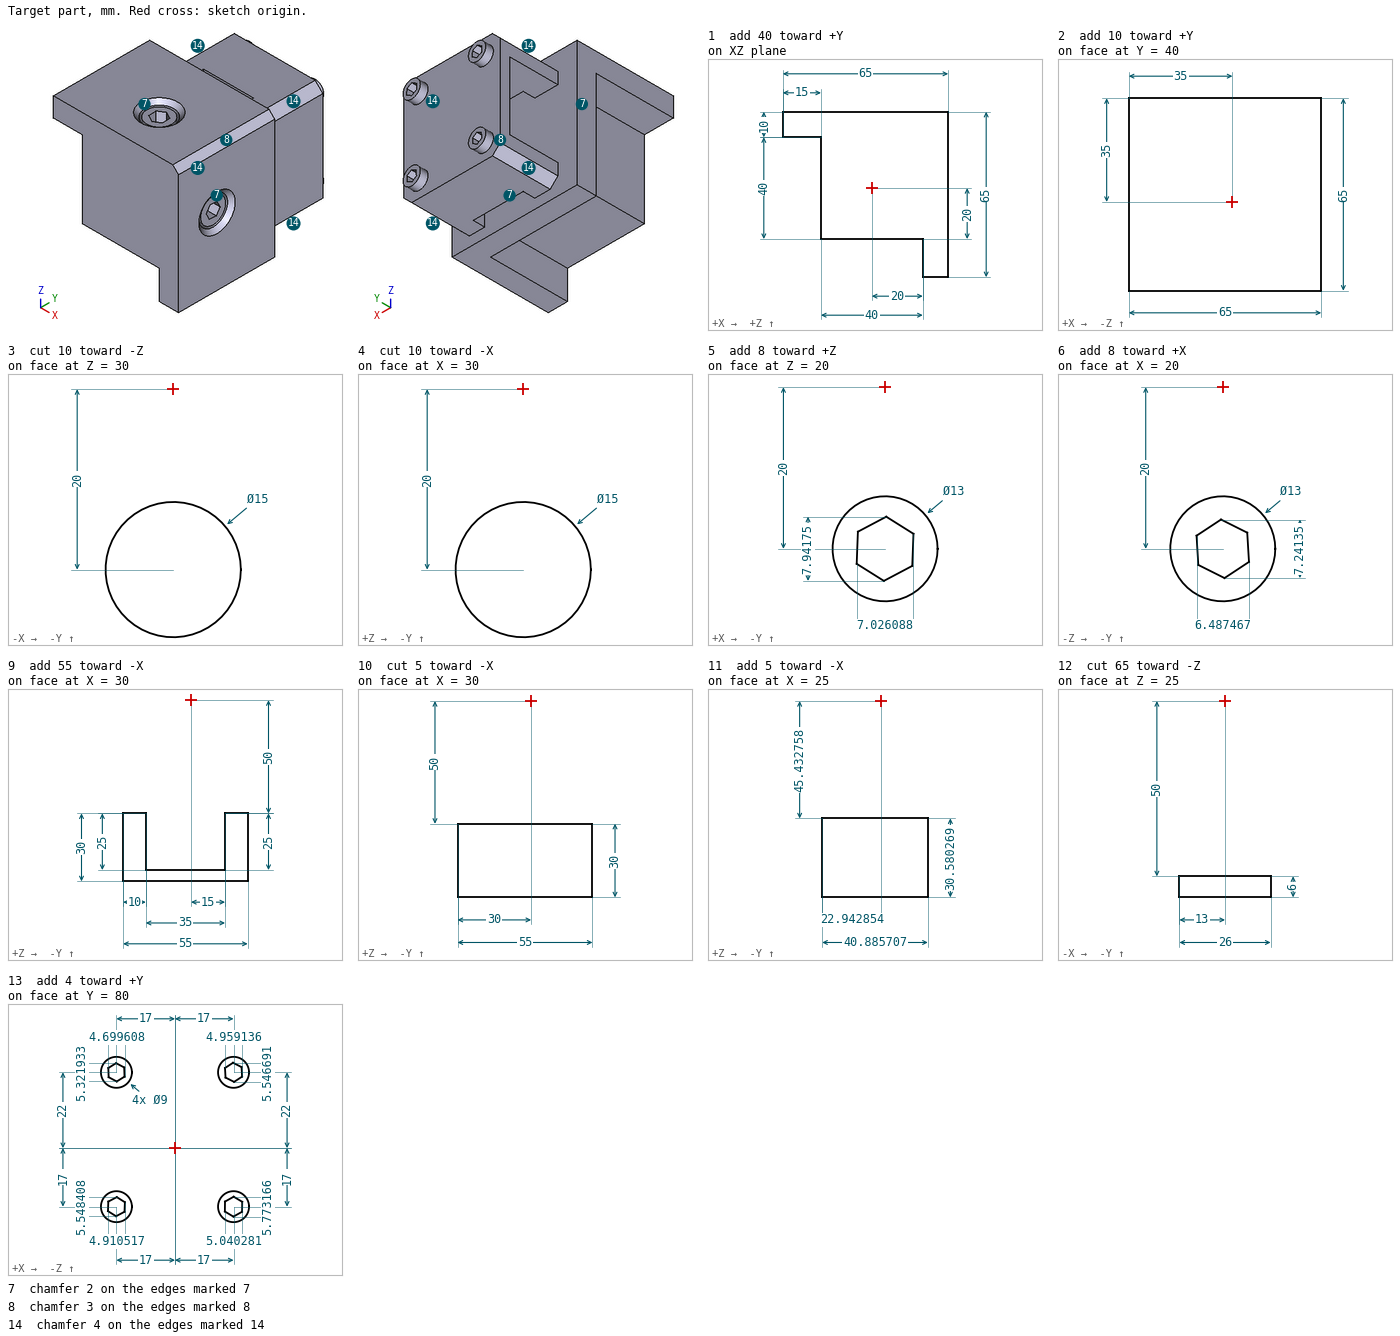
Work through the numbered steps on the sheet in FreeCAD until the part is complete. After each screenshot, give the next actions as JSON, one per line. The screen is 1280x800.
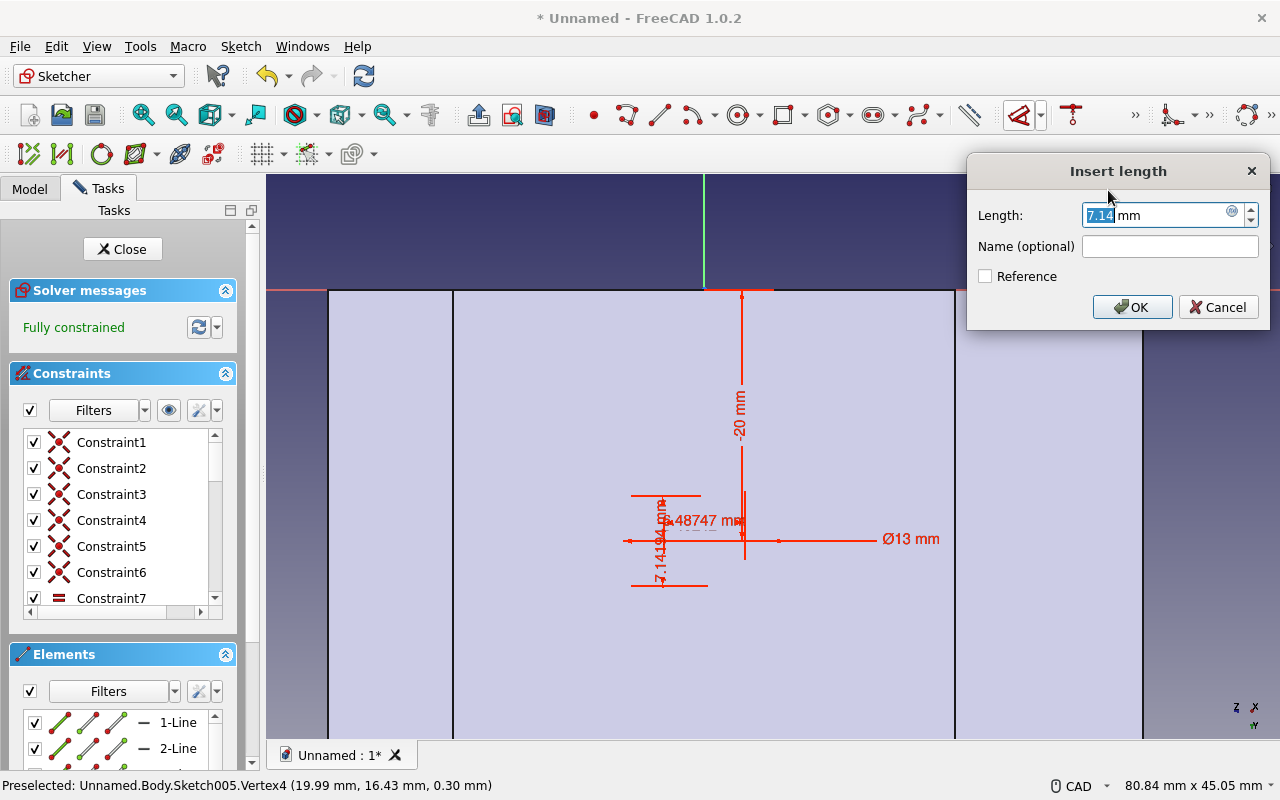
{"action": "type", "text": "7.24135"}
{"action": "key", "text": "Return"}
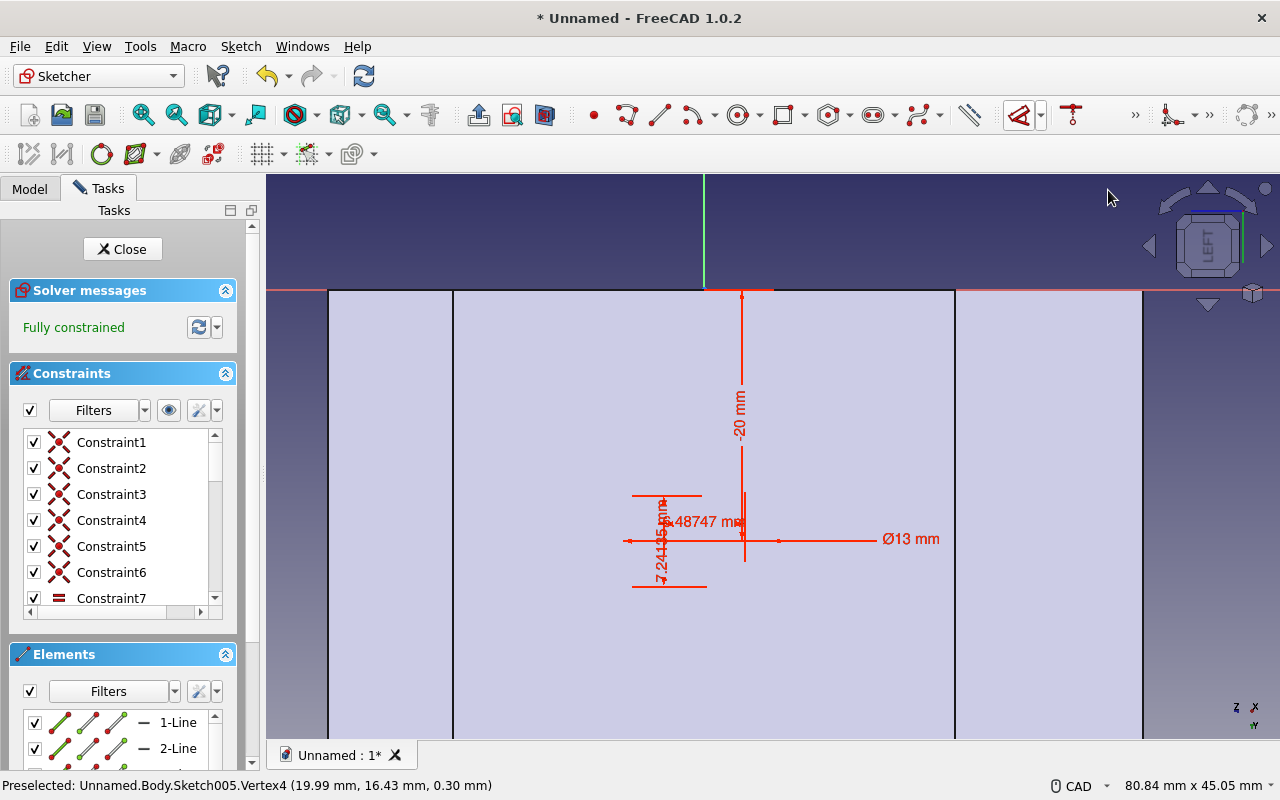
{"action": "left_click", "coordinate": [123, 249]}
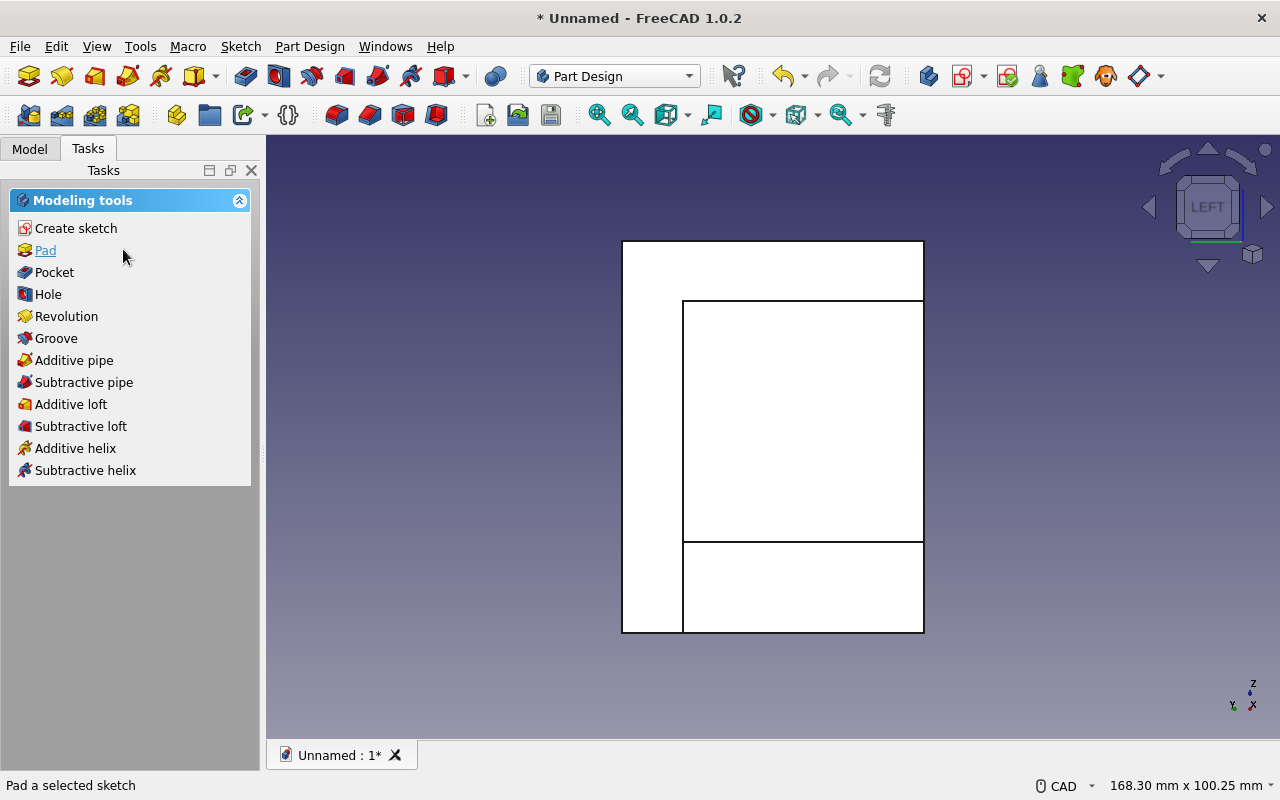
{"action": "left_click", "coordinate": [29, 76]}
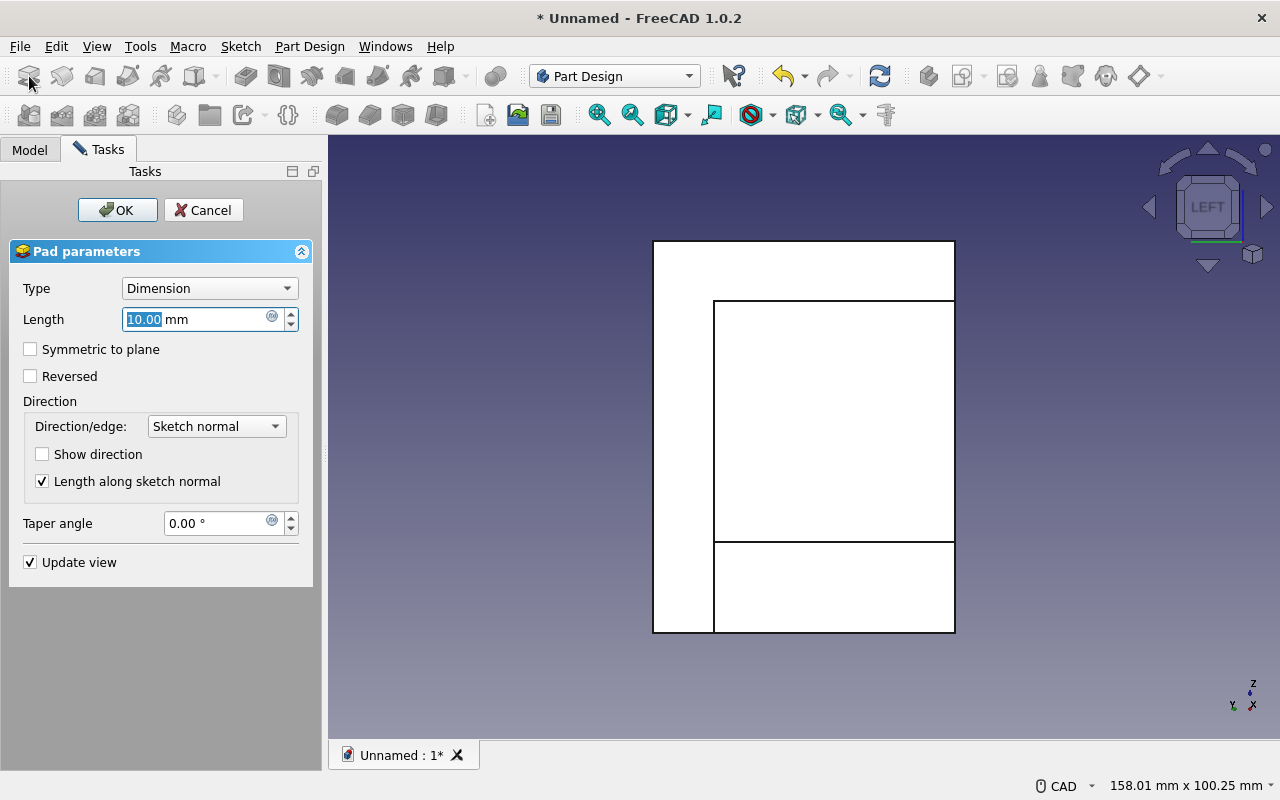
{"action": "type", "text": "8"}
{"action": "key", "text": "Tab"}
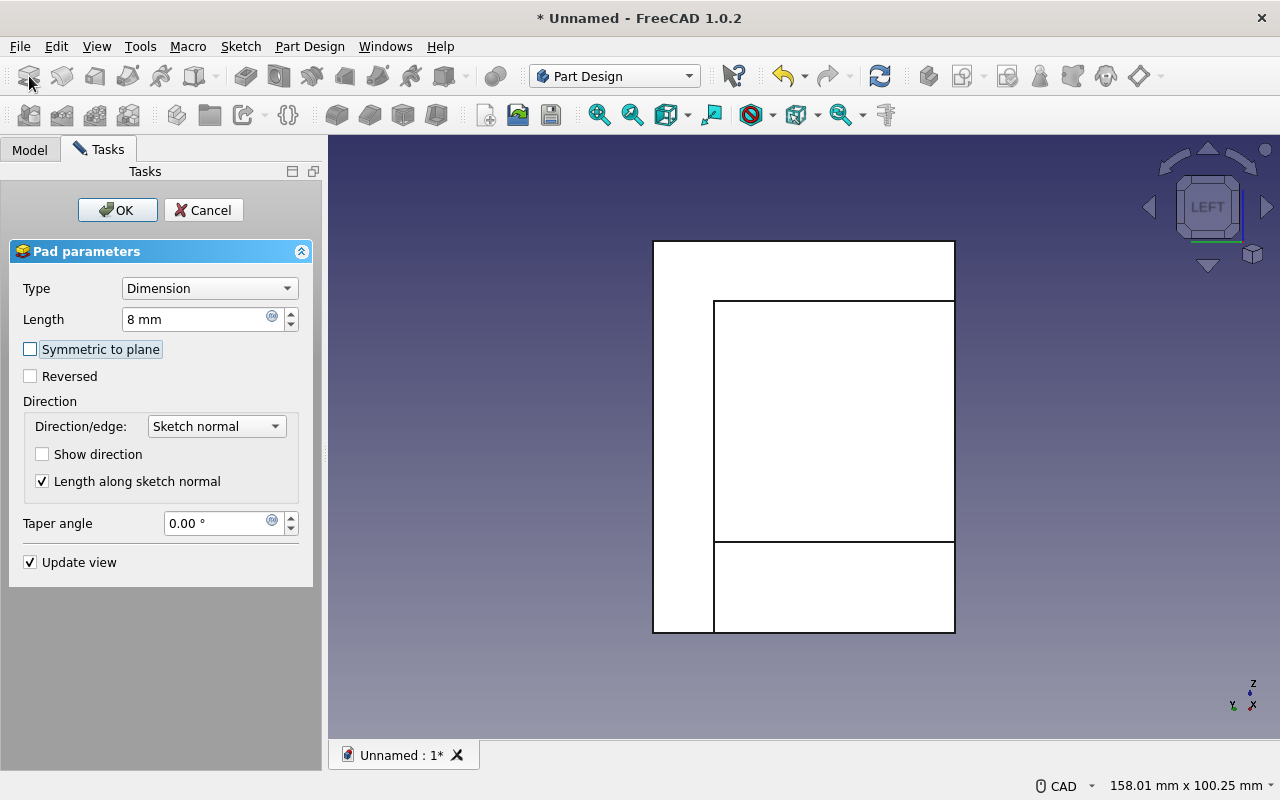
{"action": "left_click", "coordinate": [31, 376]}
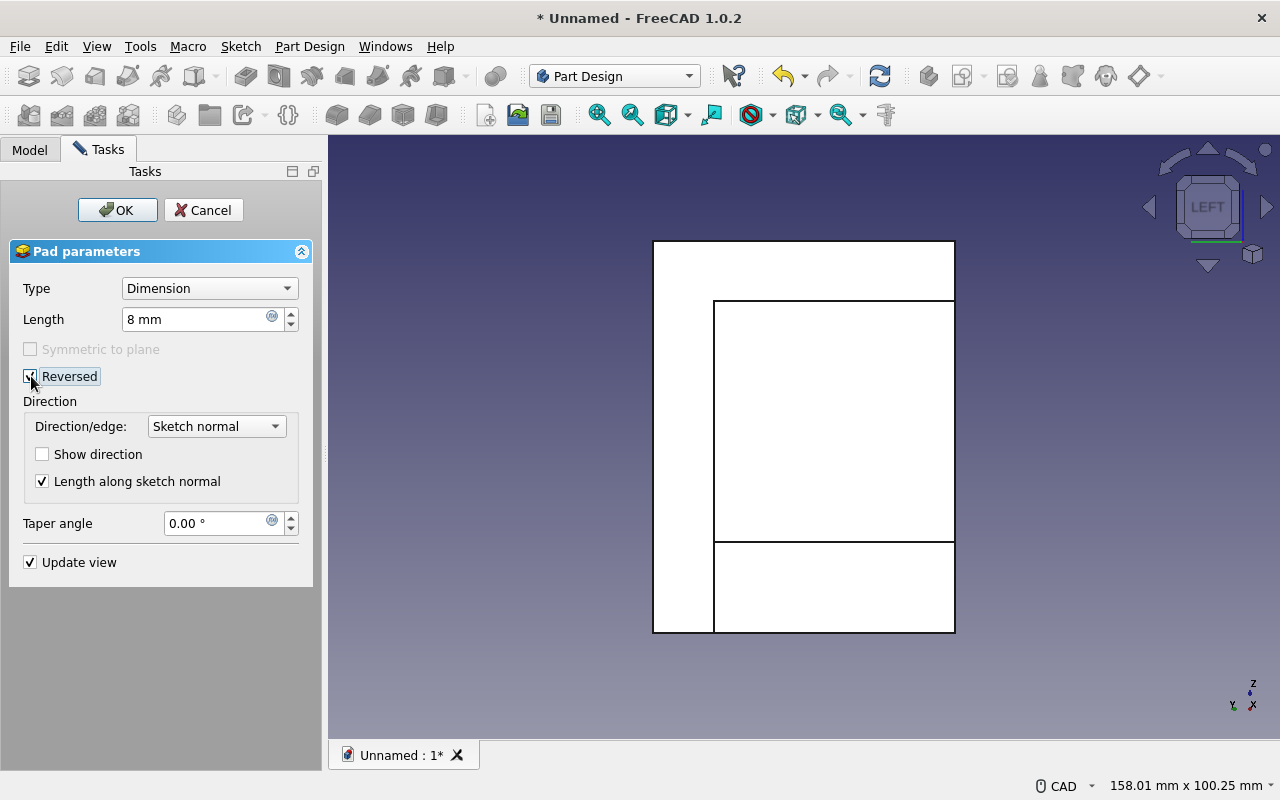
{"action": "left_click", "coordinate": [118, 210]}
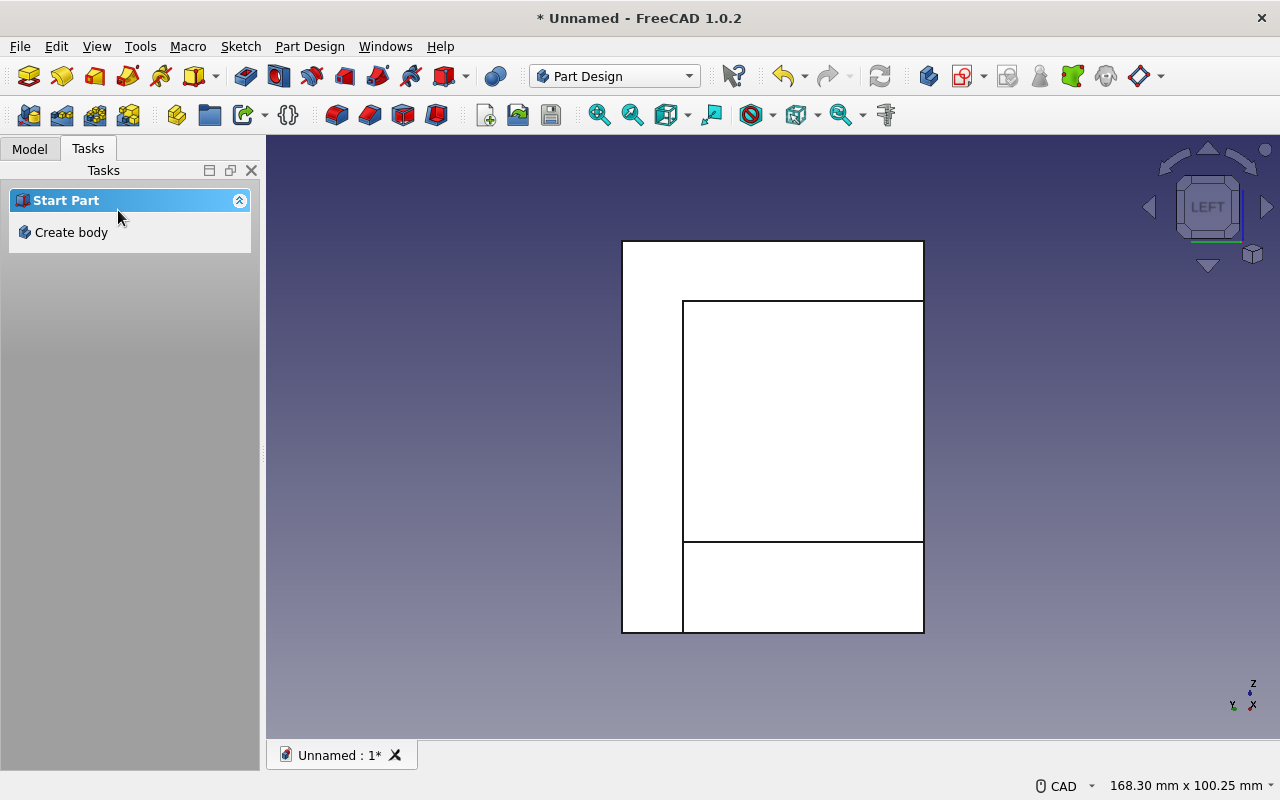
{"action": "key", "text": "0"}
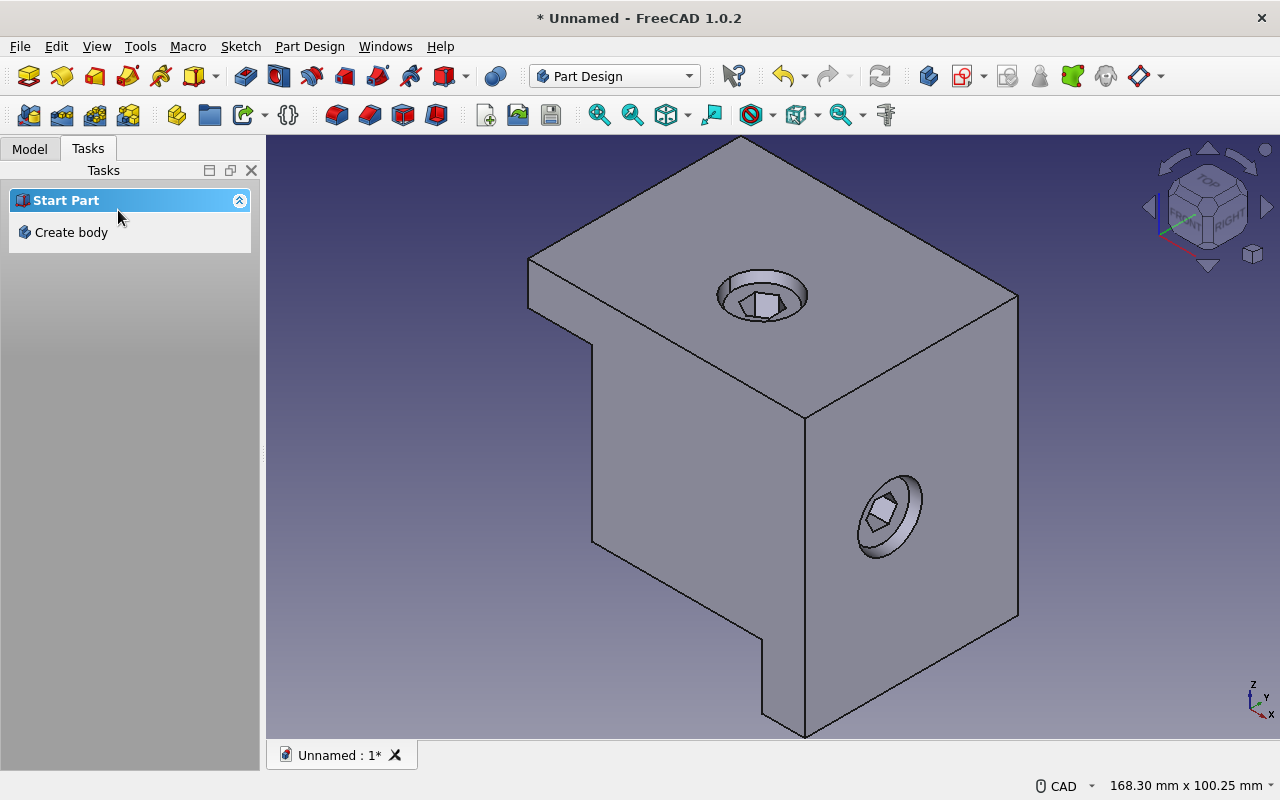
{"action": "left_click", "coordinate": [803, 283]}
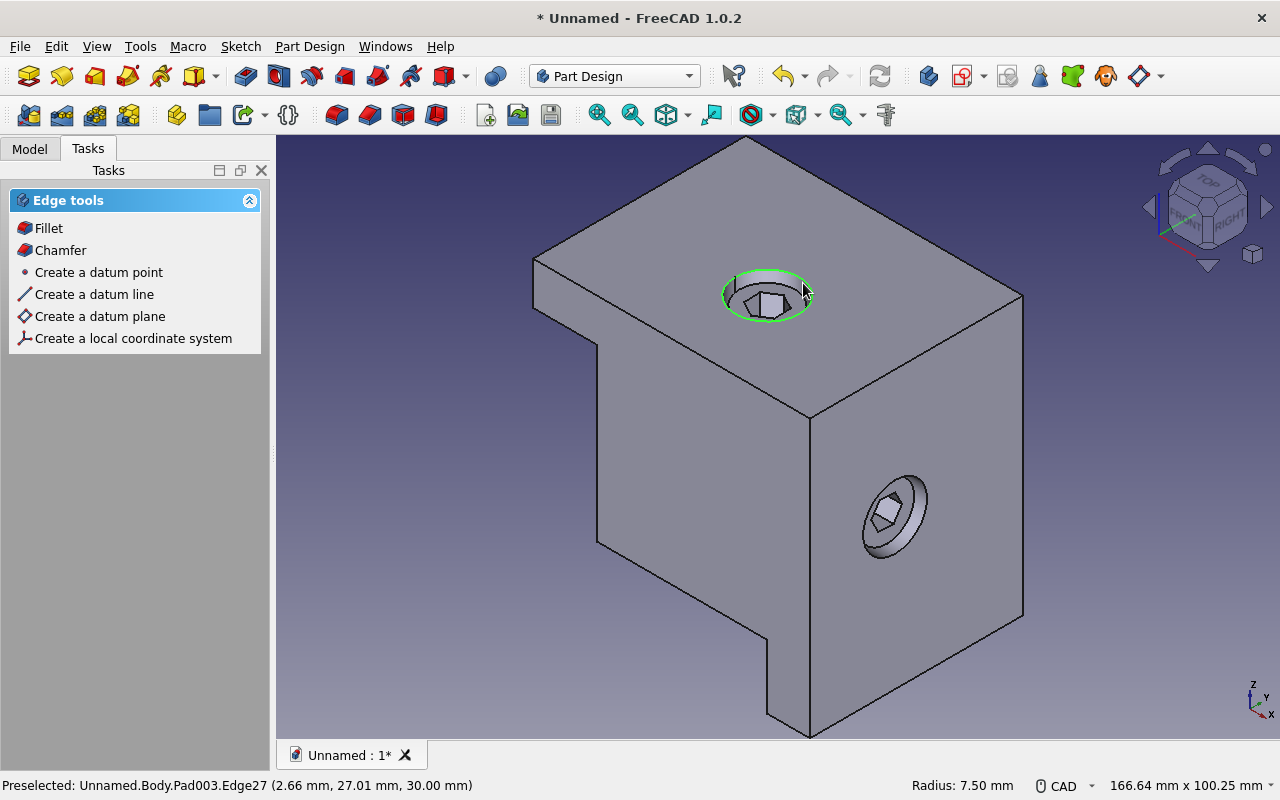
{"action": "left_click", "coordinate": [895, 553], "text": "ctrl"}